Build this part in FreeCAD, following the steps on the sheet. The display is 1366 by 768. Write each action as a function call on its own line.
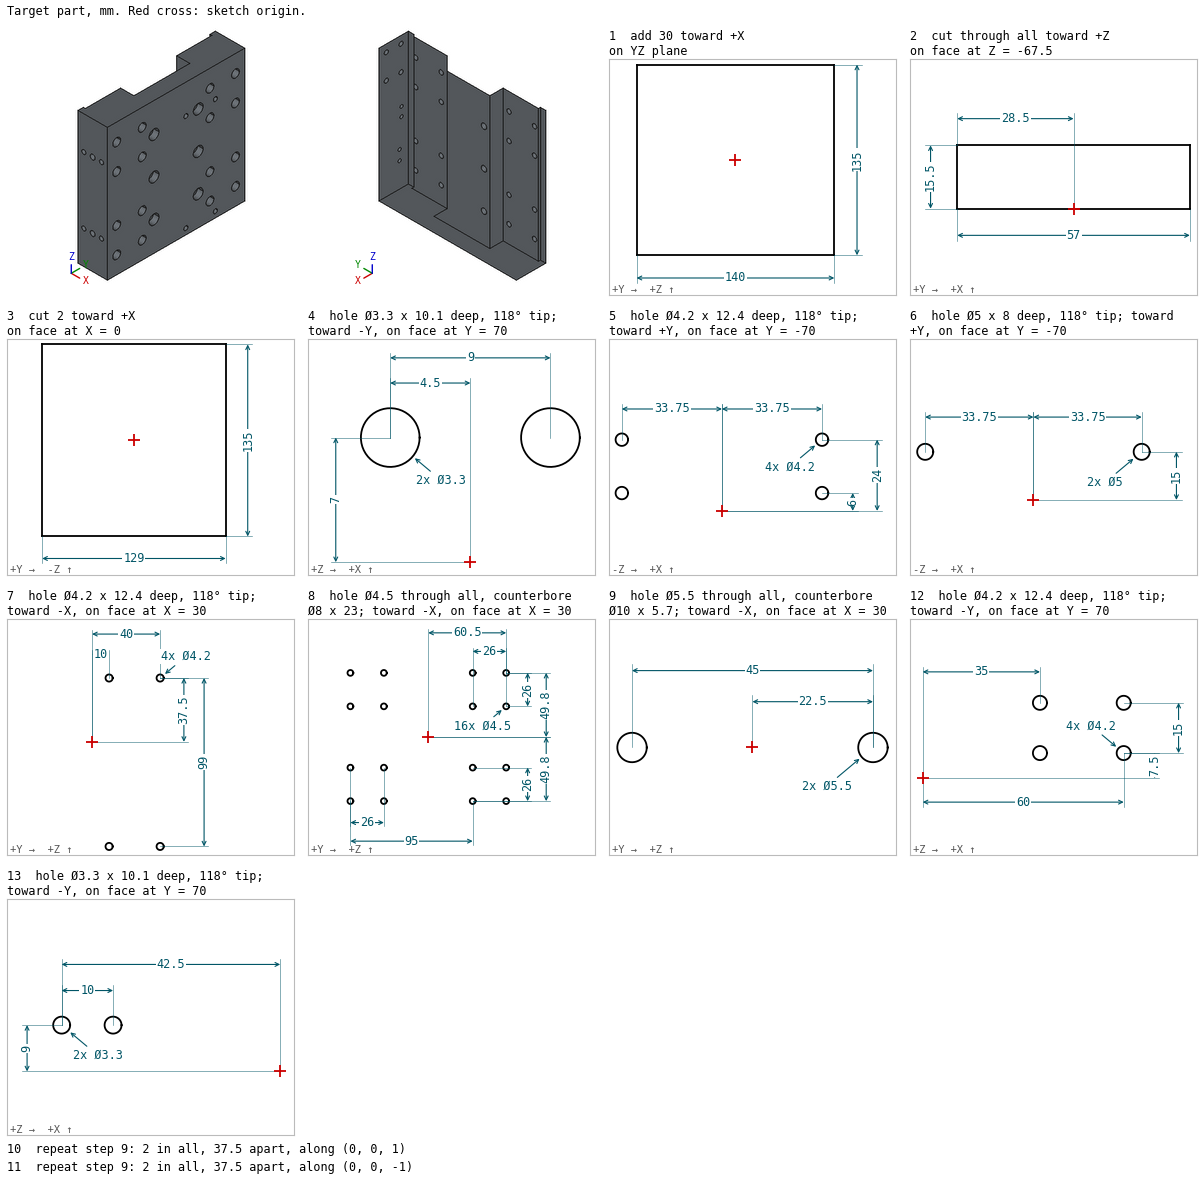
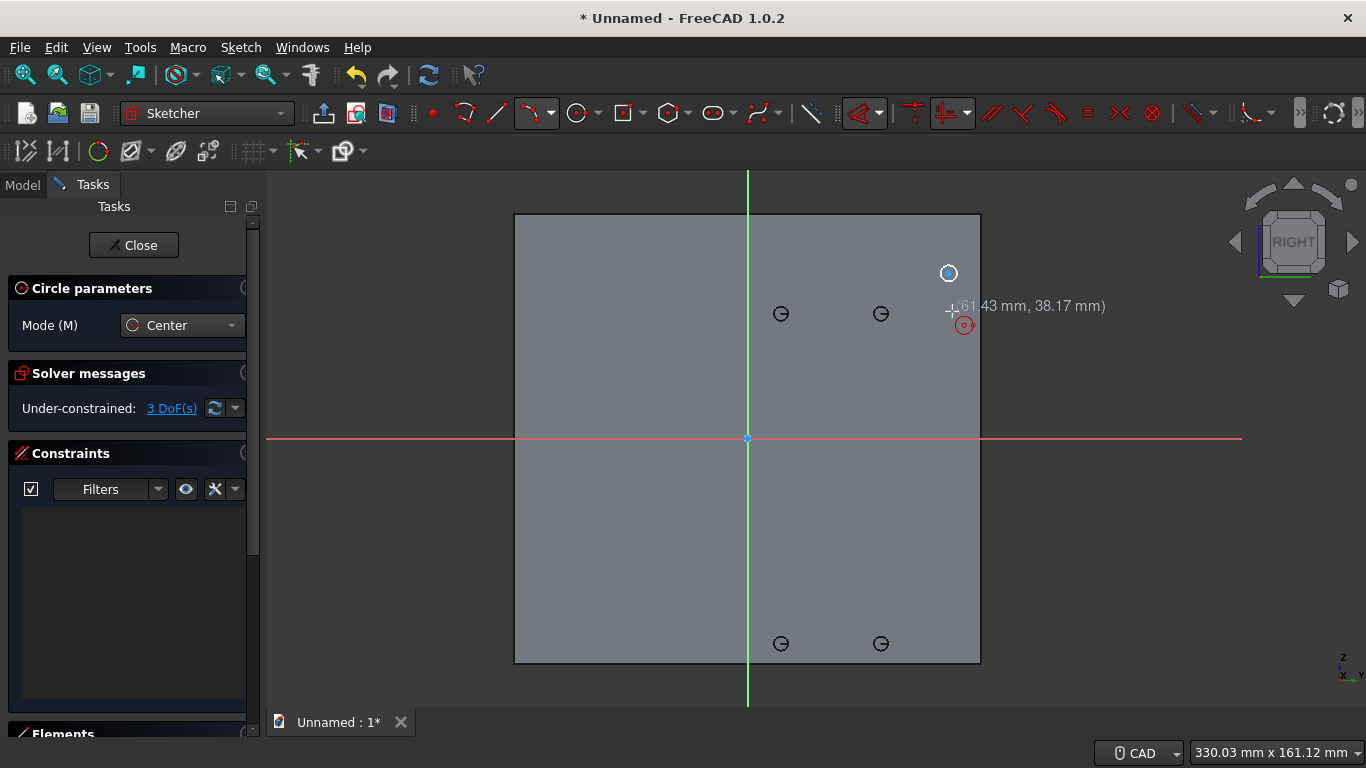
click(949, 359)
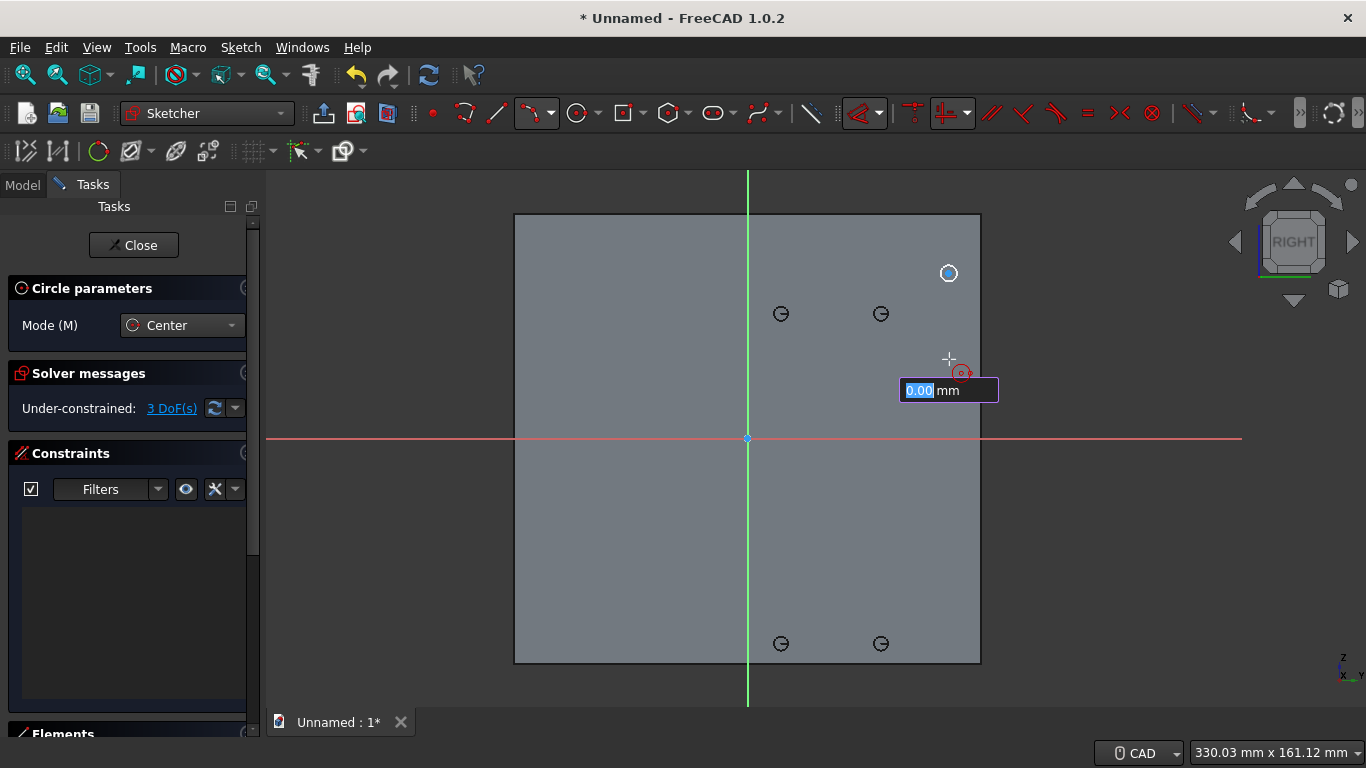
scroll(955, 354, up, 4)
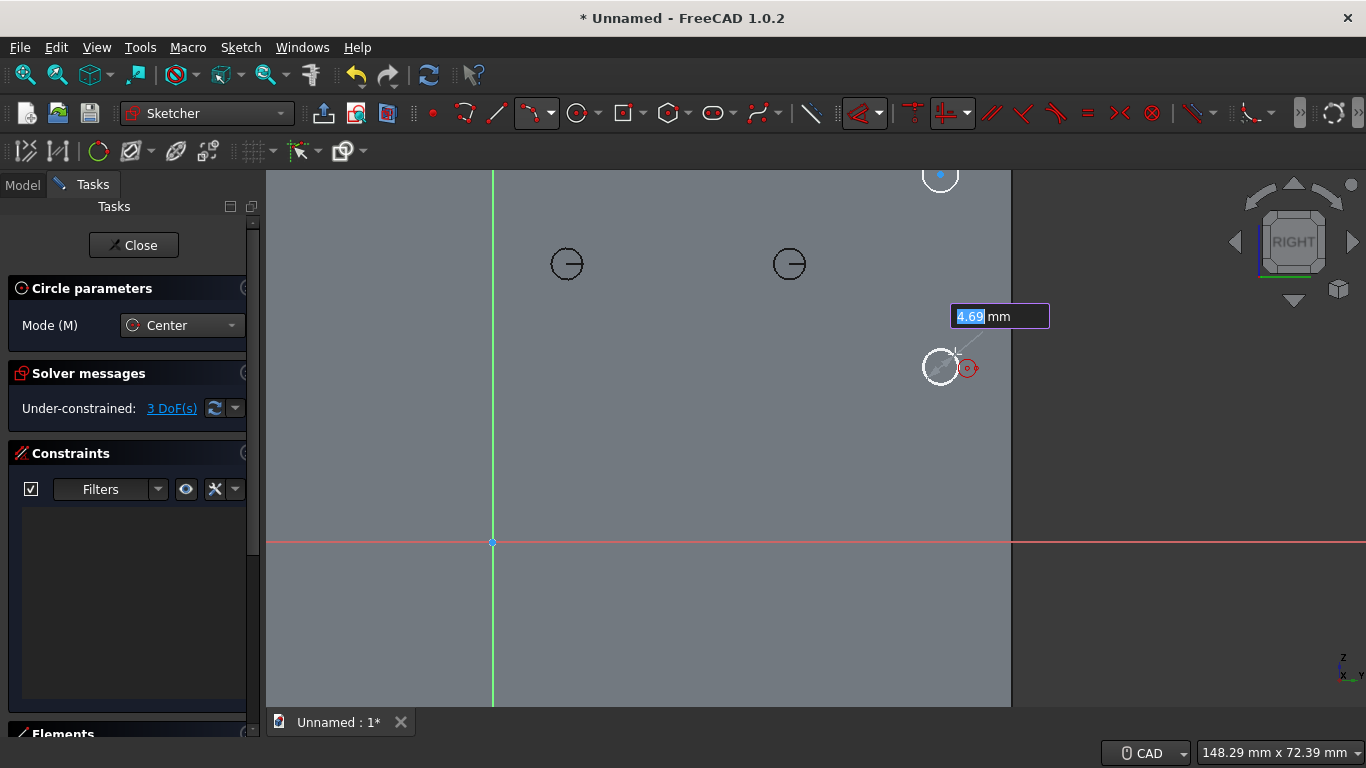
click(953, 354)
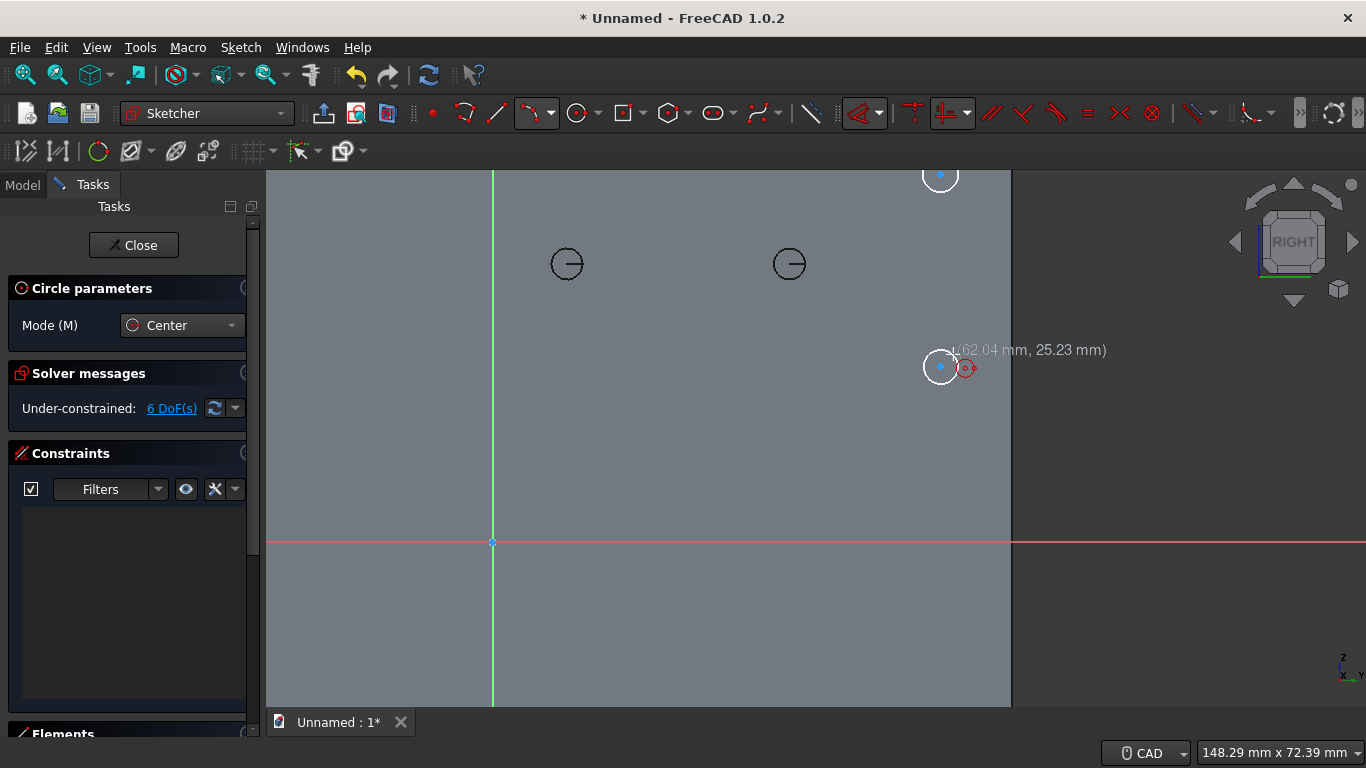
scroll(749, 366, up, 2)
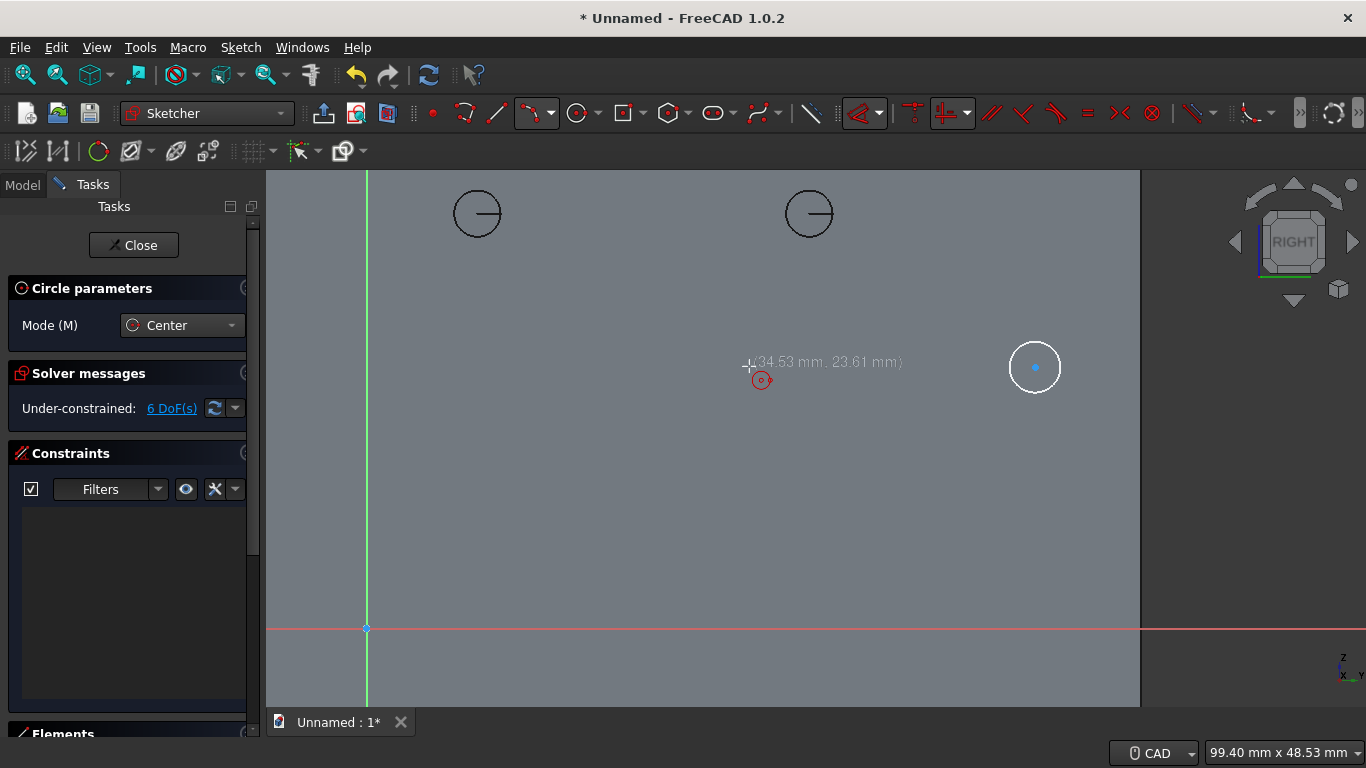
scroll(912, 357, down, 6)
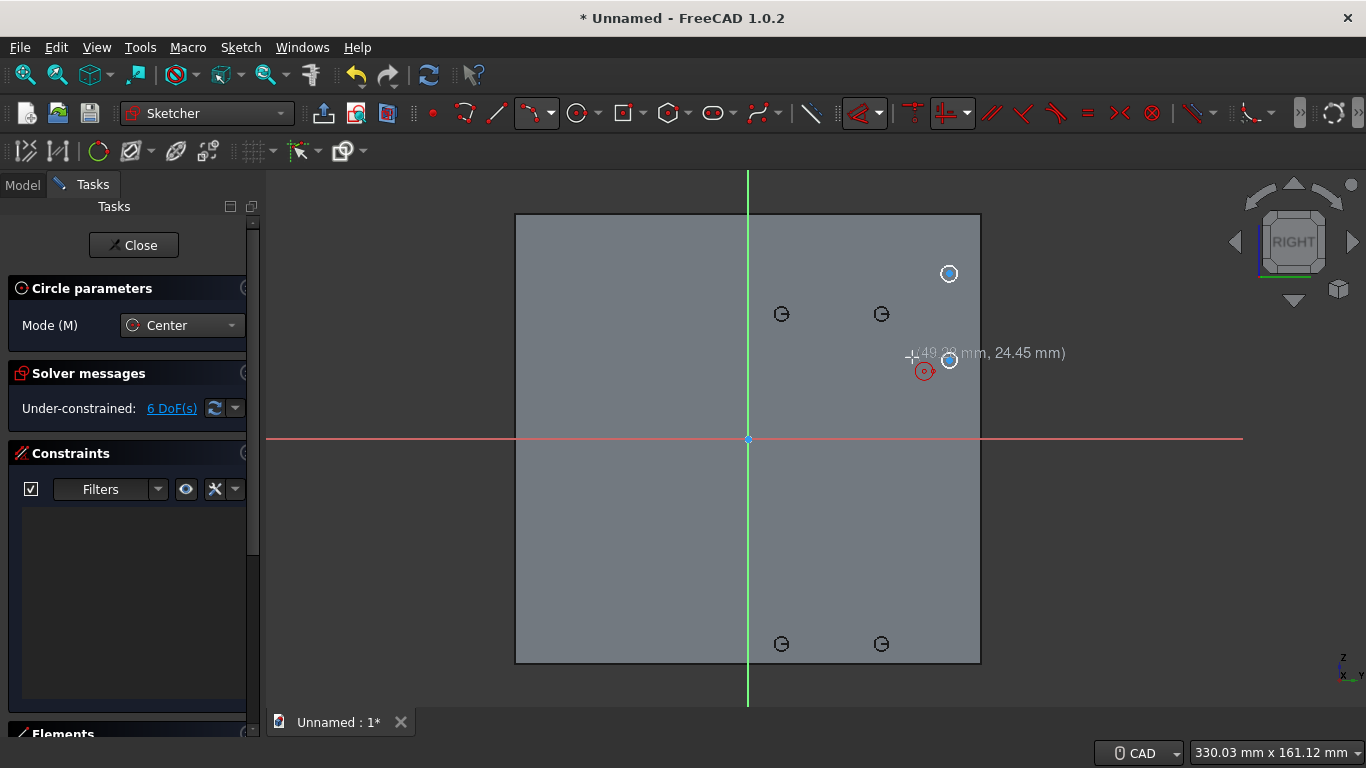
click(863, 360)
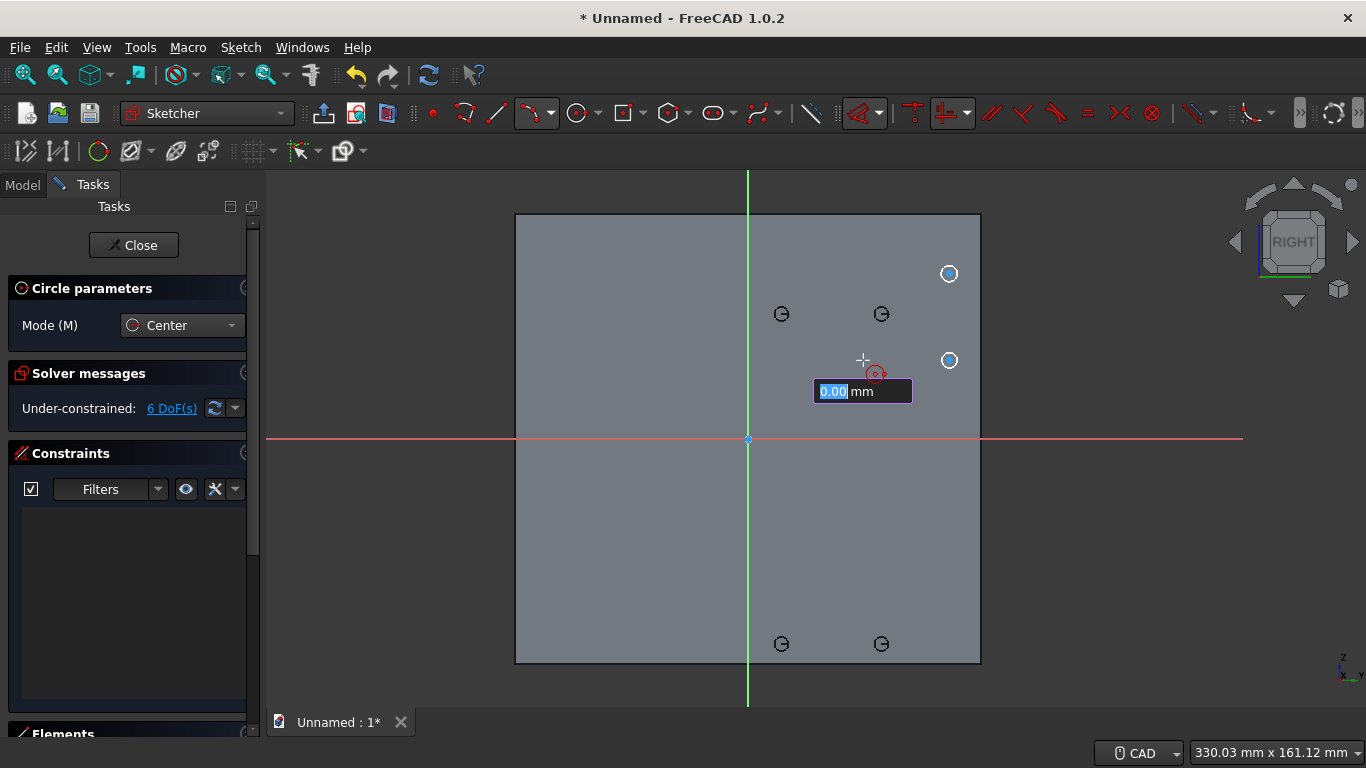
scroll(868, 354, up, 4)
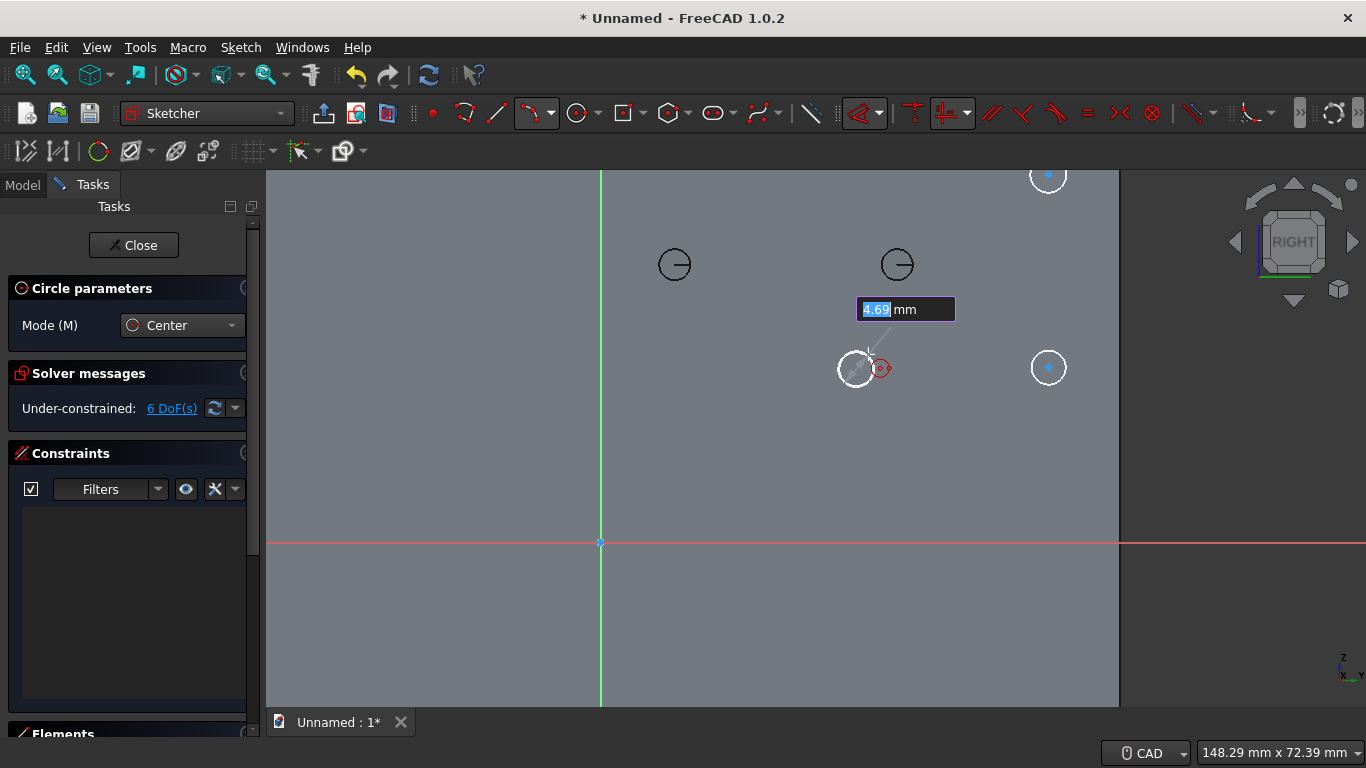
click(868, 354)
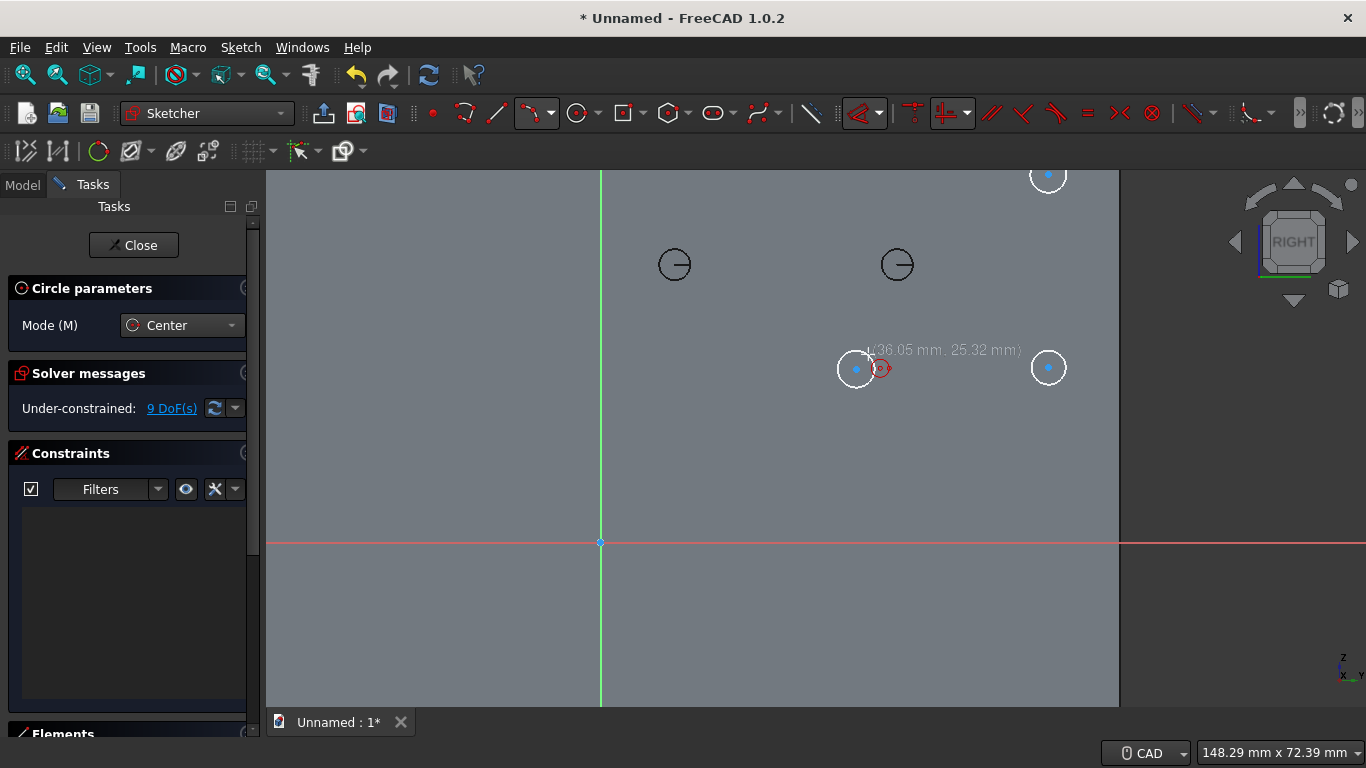
scroll(867, 353, down, 4)